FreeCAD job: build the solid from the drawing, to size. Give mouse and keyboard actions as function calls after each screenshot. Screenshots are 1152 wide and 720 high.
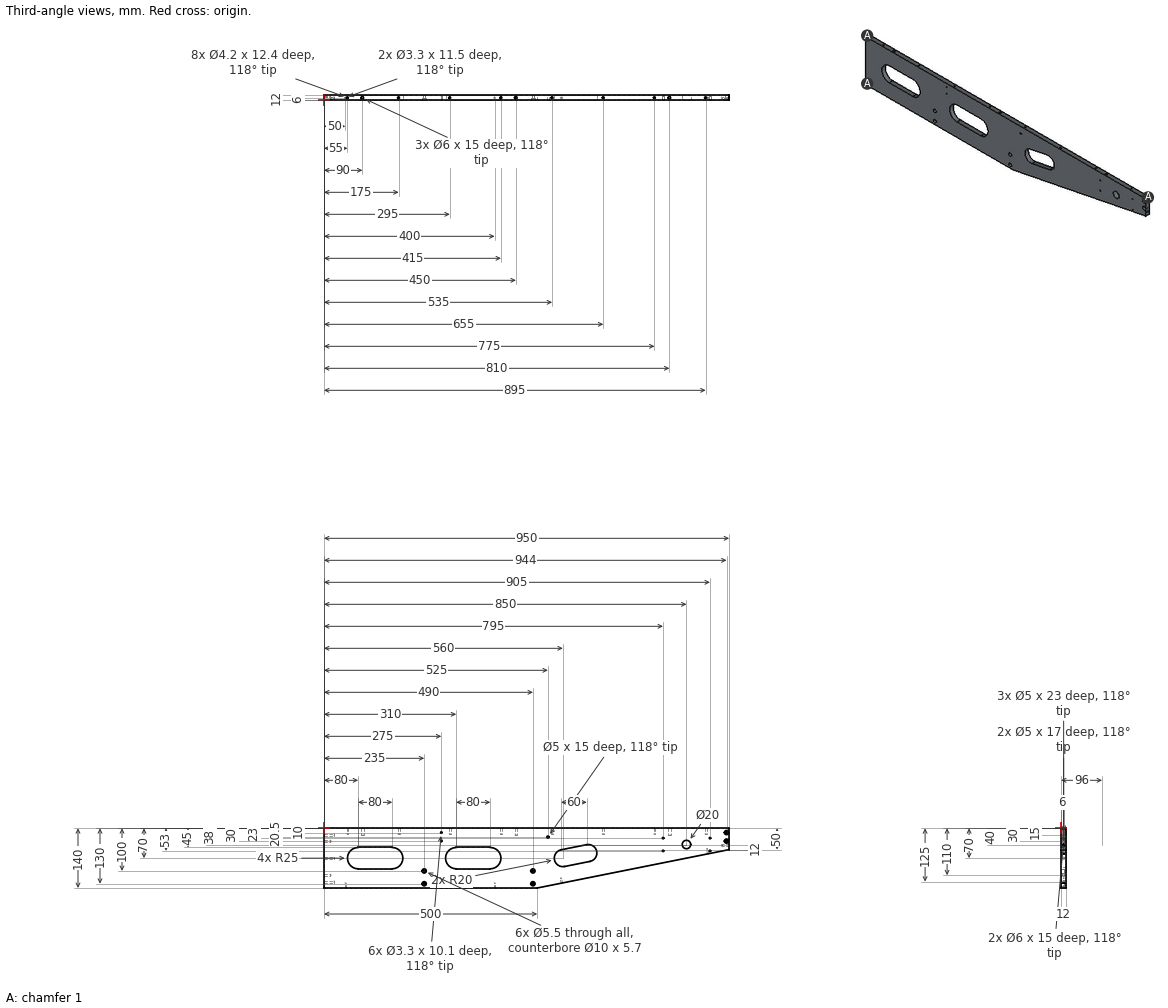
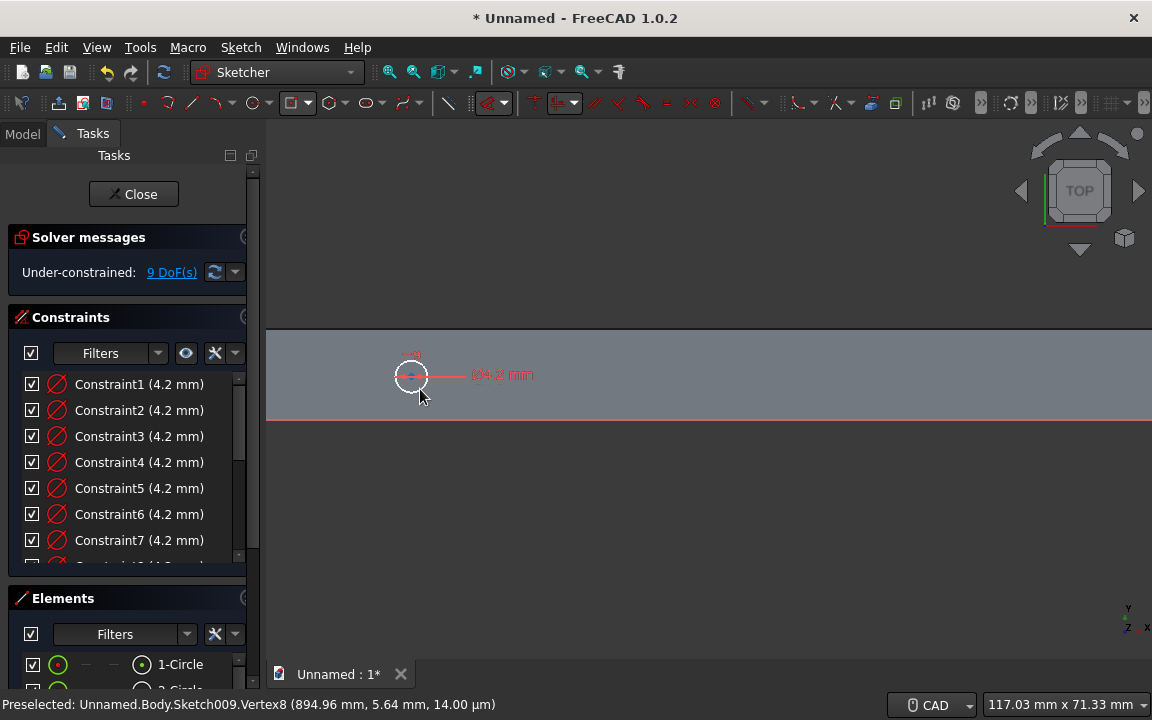
click(411, 377)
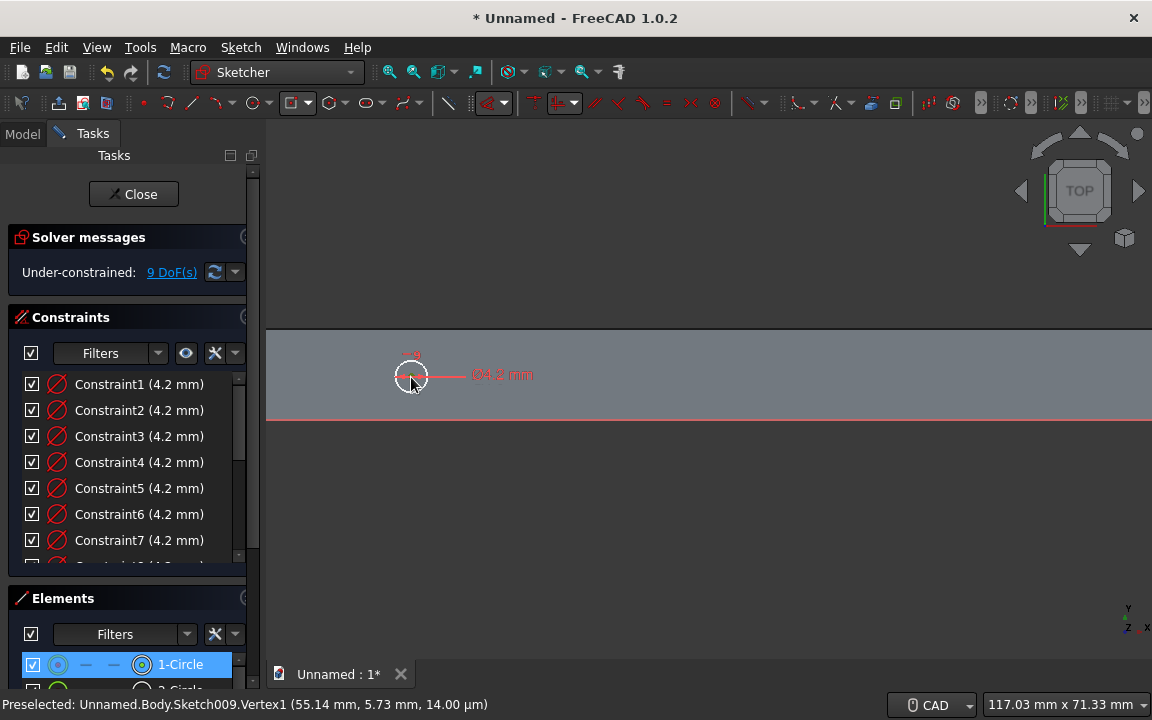
click(506, 104)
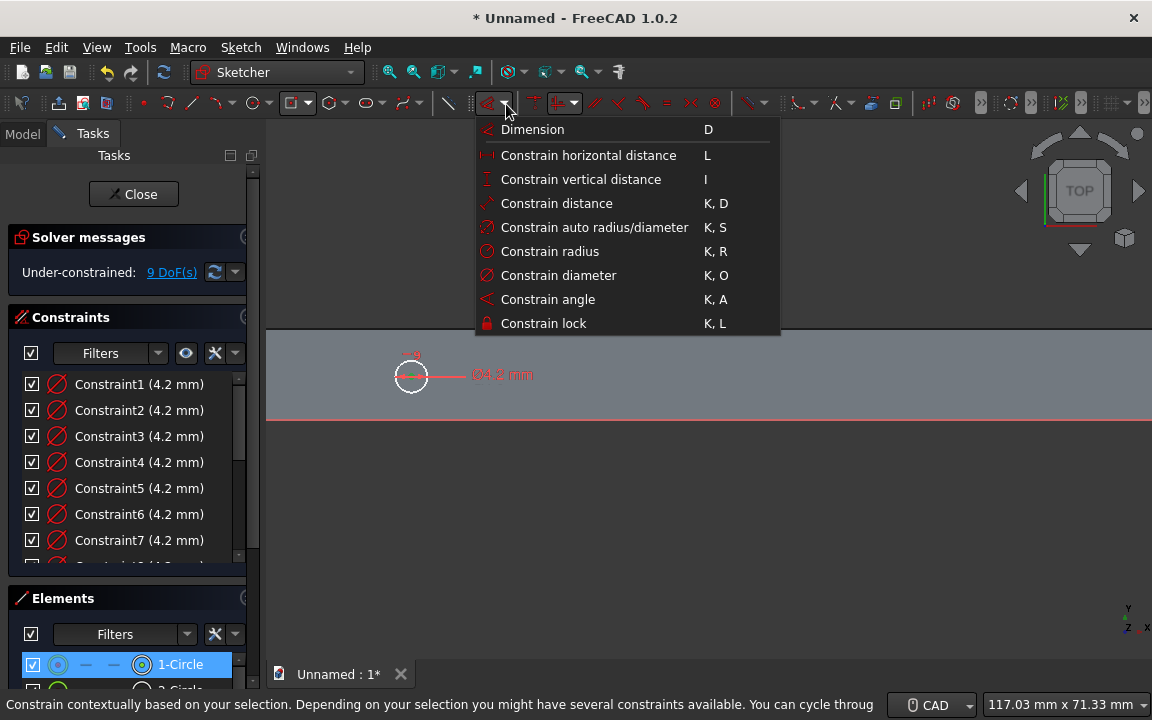
click(628, 179)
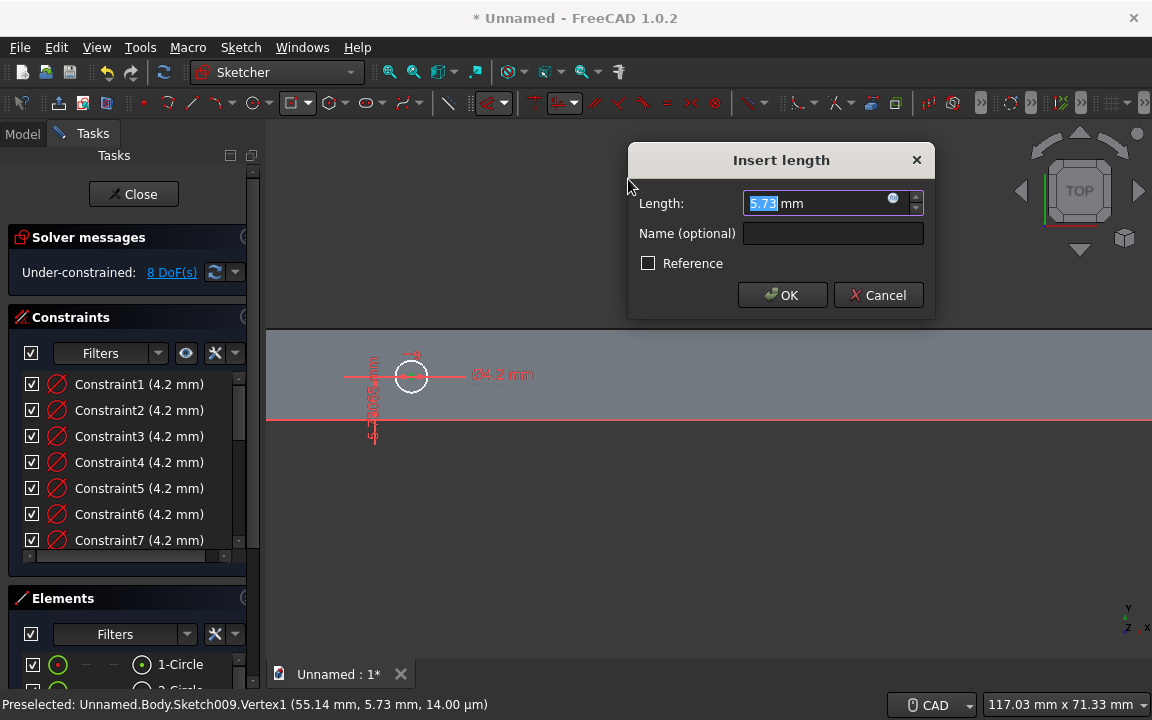
text(6)
key(Return)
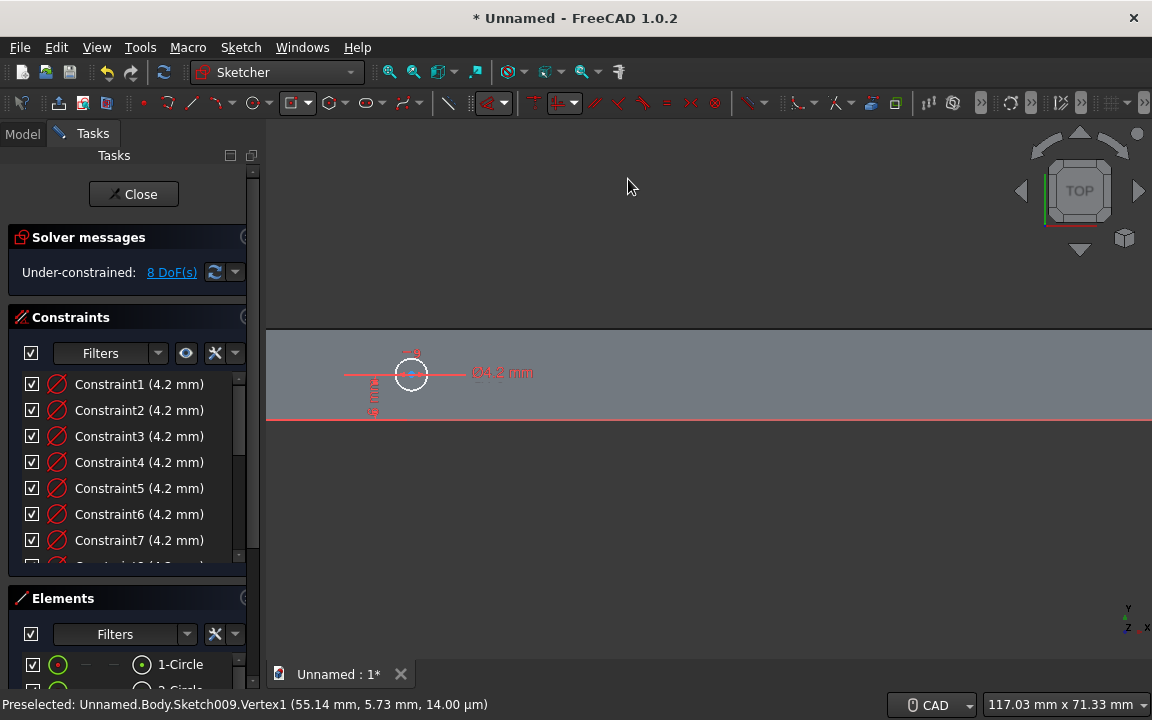
scroll(420, 389, down, 13)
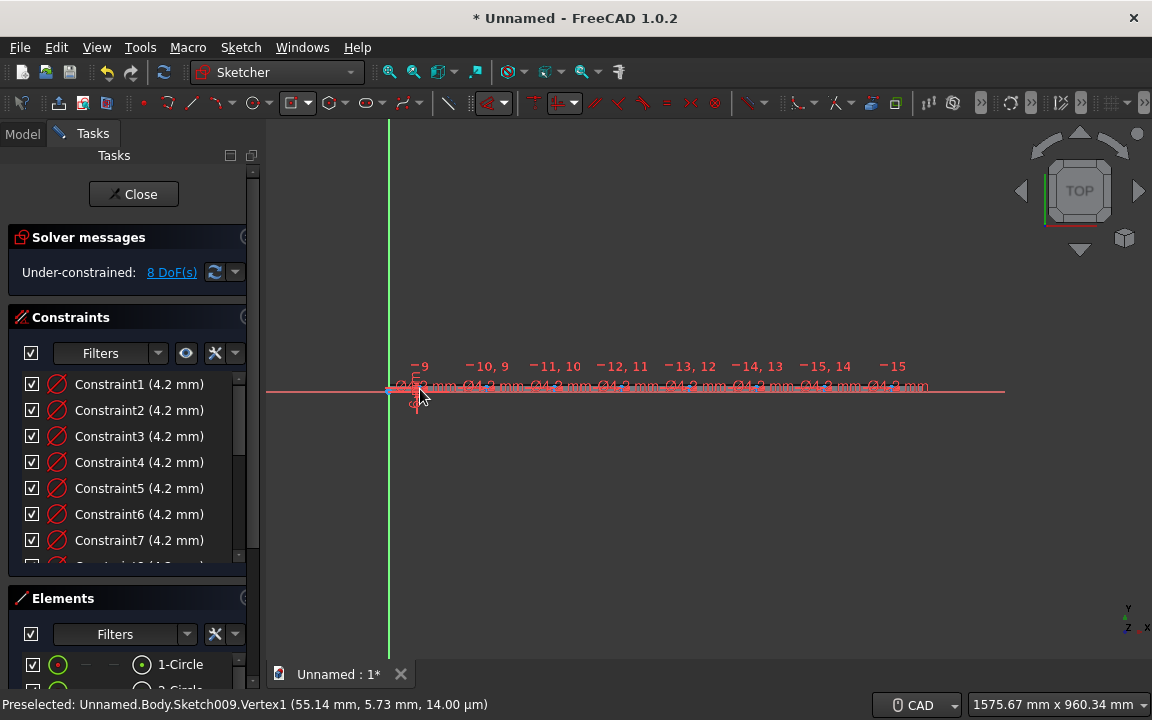
scroll(420, 388, up, 2)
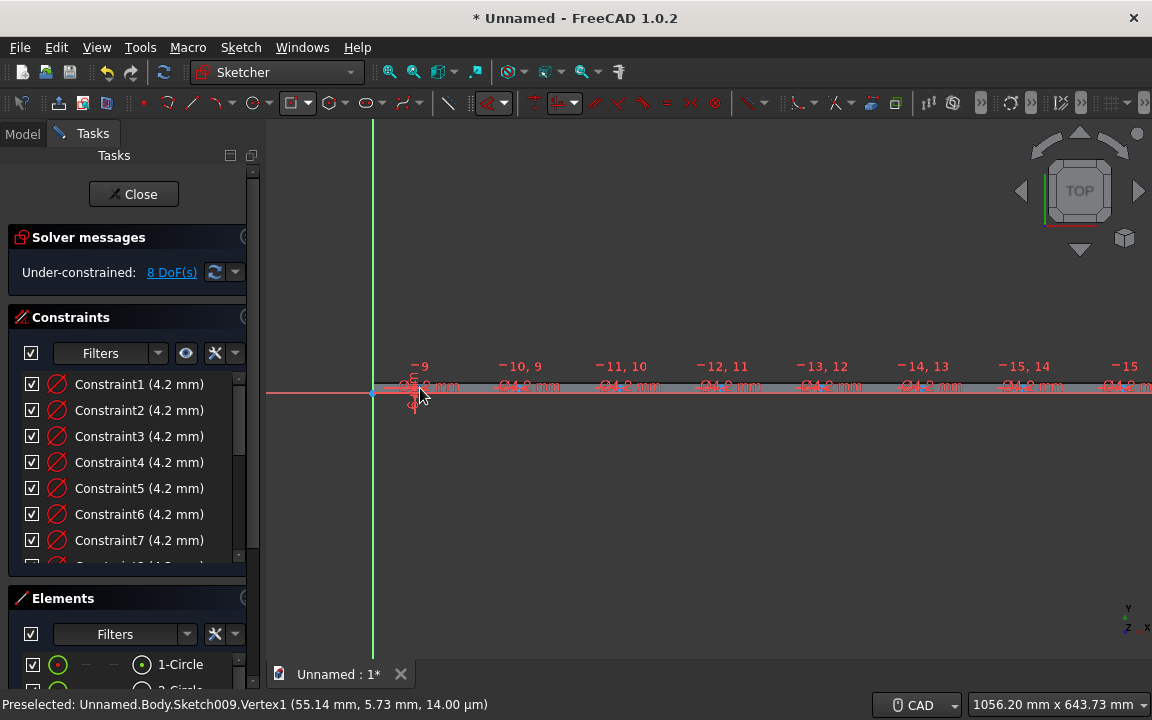
click(419, 388)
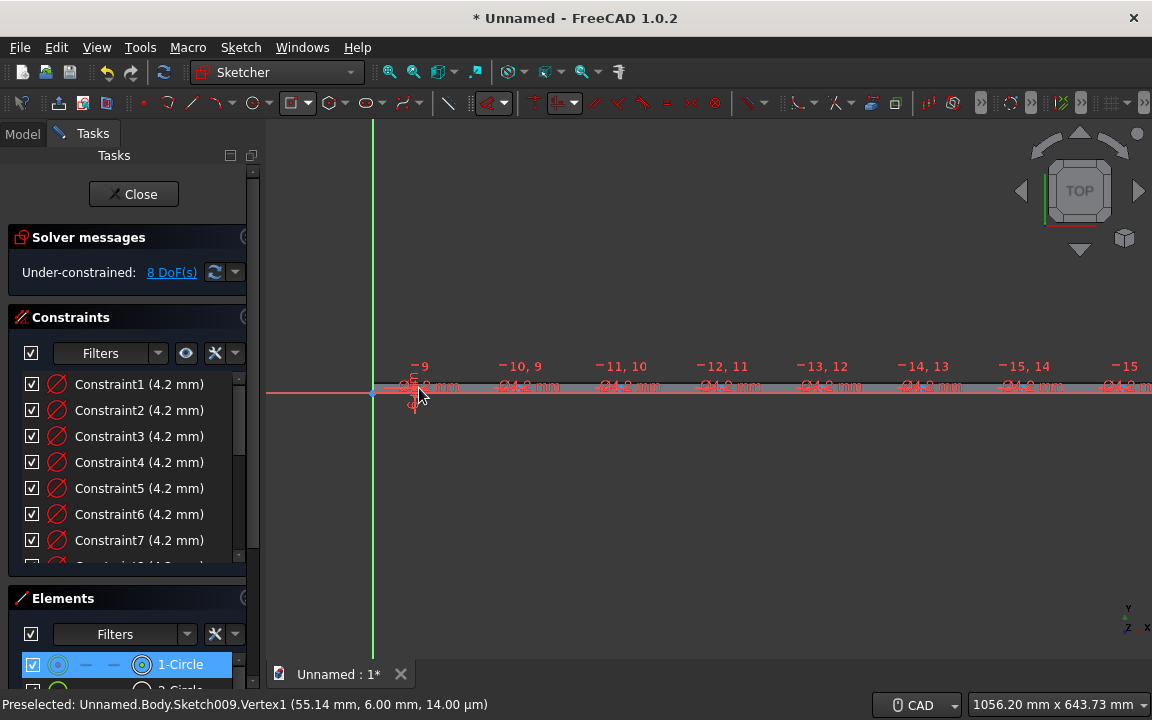
click(506, 104)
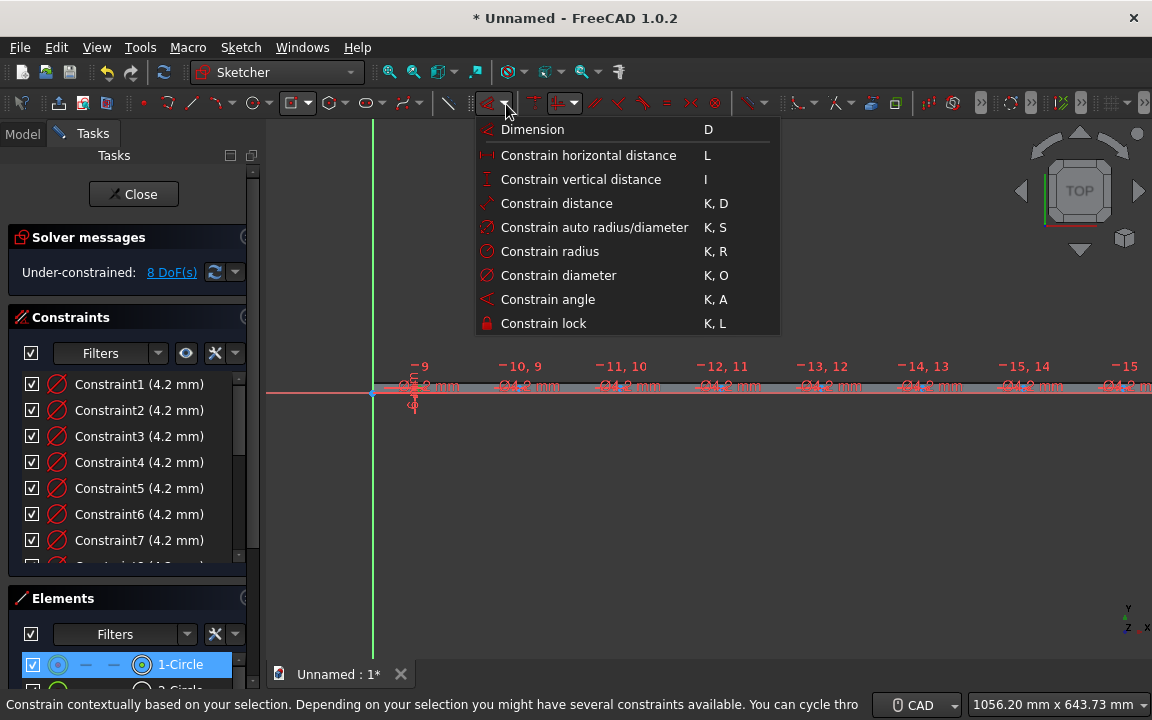
click(628, 155)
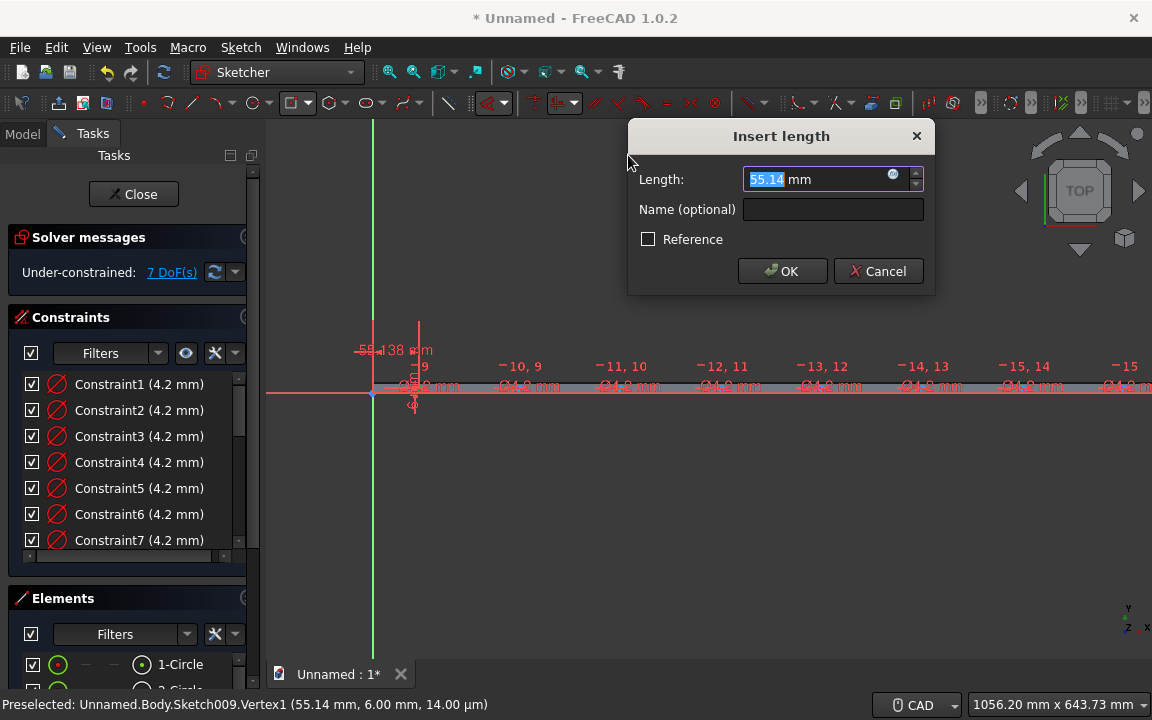
text(55)
key(Return)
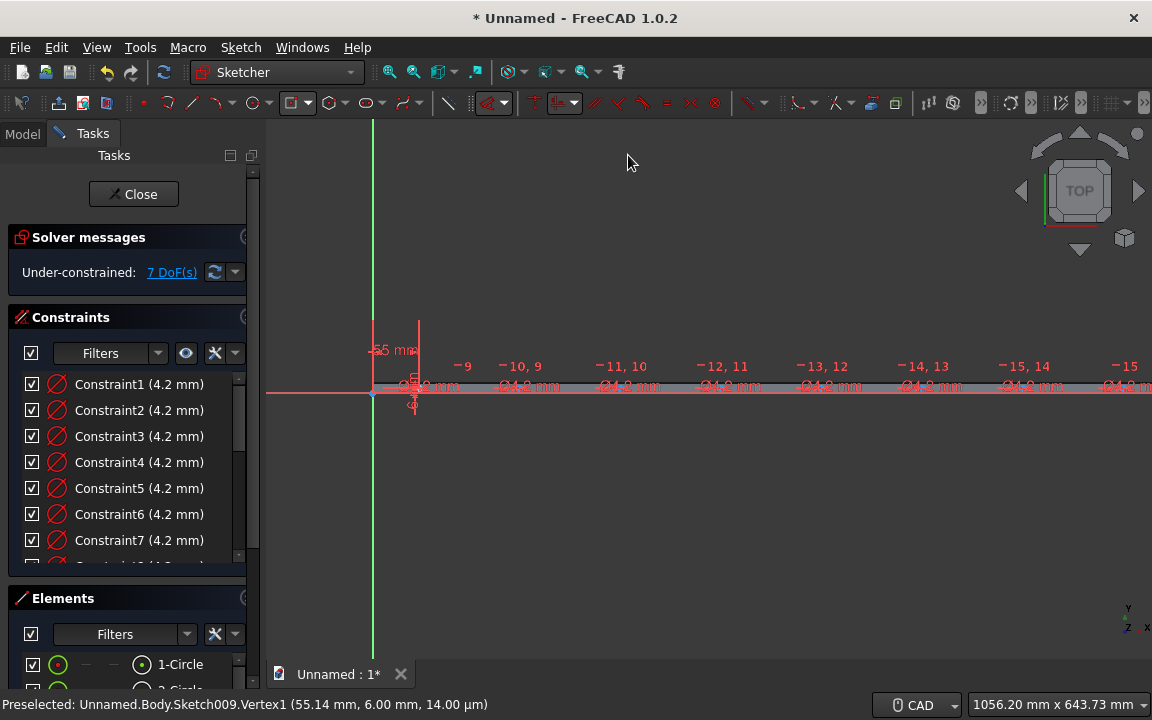
click(520, 388)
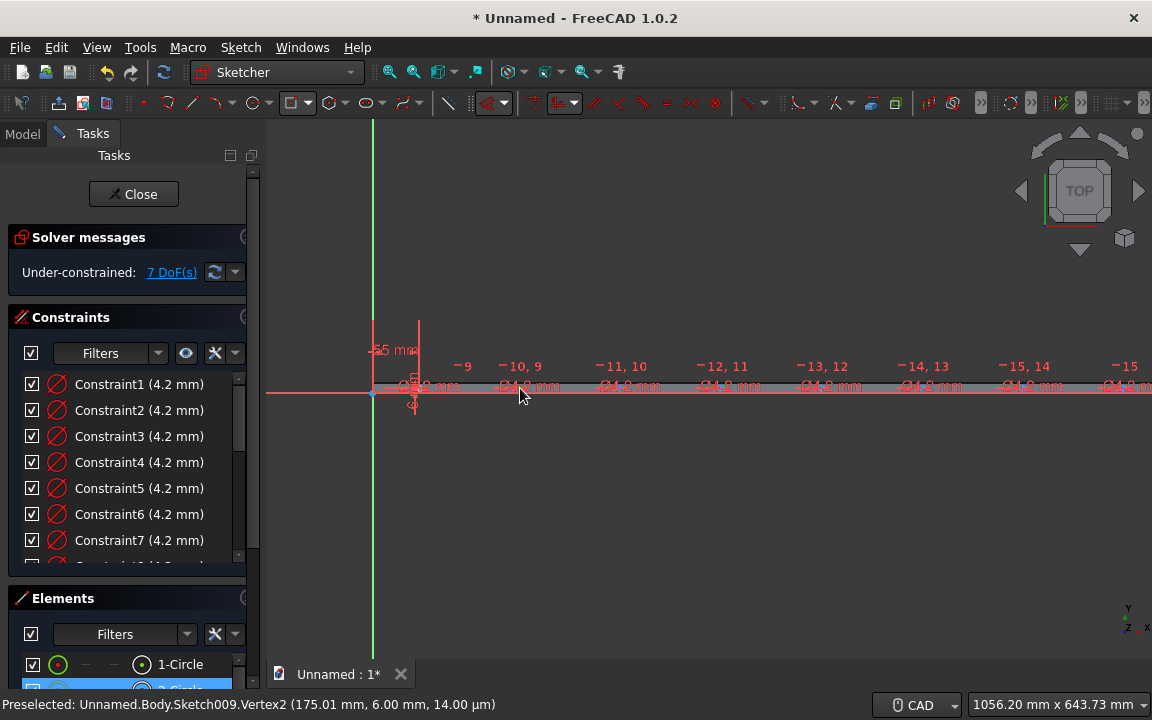
key(l)